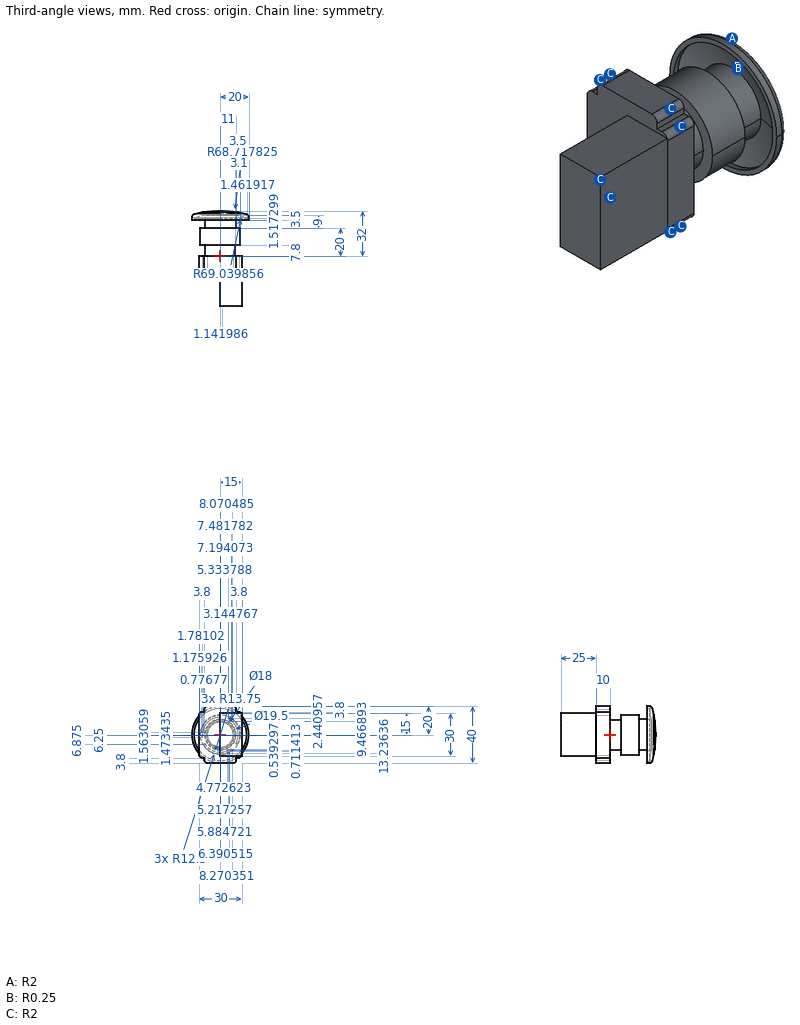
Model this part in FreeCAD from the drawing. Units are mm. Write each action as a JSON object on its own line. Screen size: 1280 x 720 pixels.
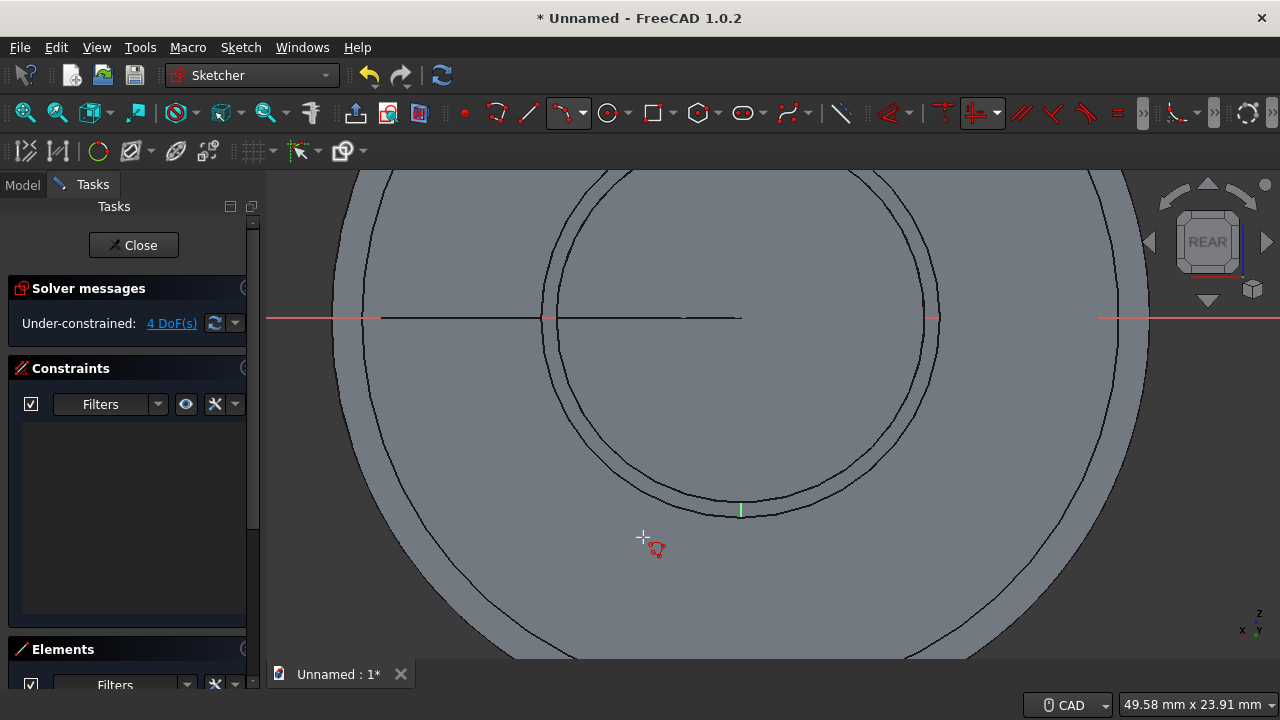
{"action": "left_click", "coordinate": [643, 536]}
{"action": "left_click", "coordinate": [571, 525]}
{"action": "left_click", "coordinate": [610, 589]}
{"action": "left_click", "coordinate": [620, 573]}
{"action": "right_click", "coordinate": [620, 573]}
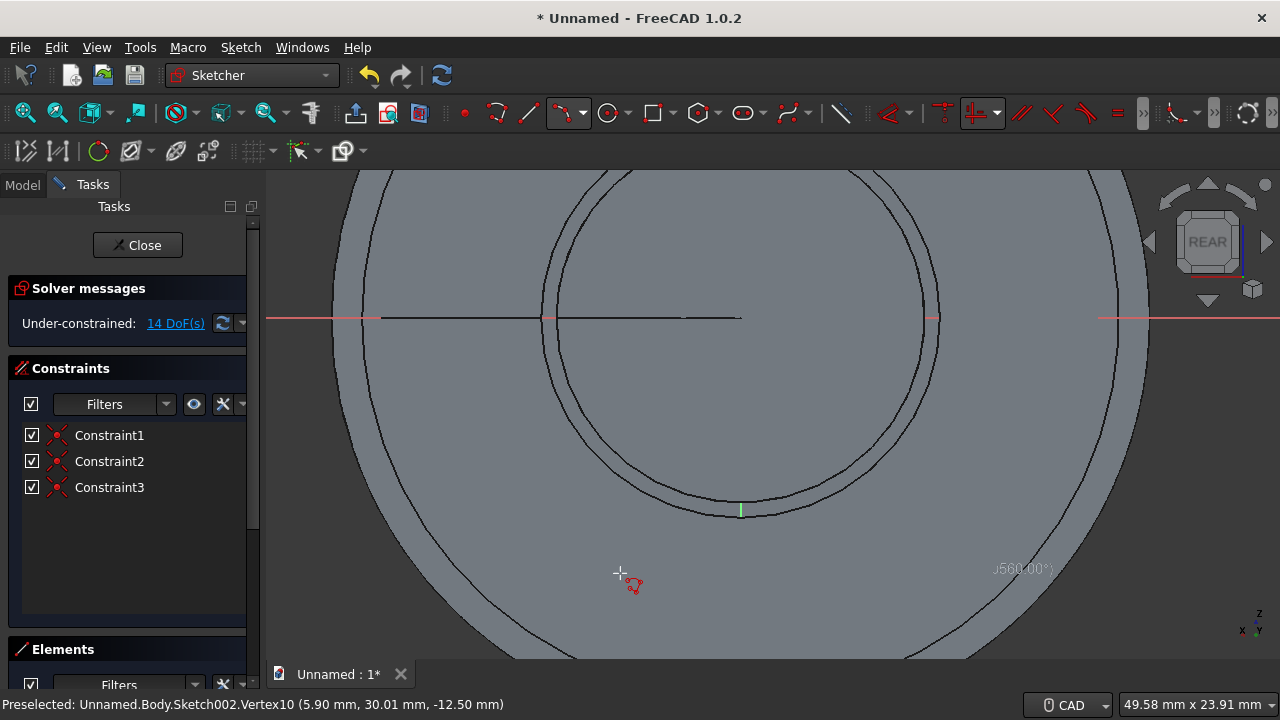
{"action": "left_click", "coordinate": [562, 114]}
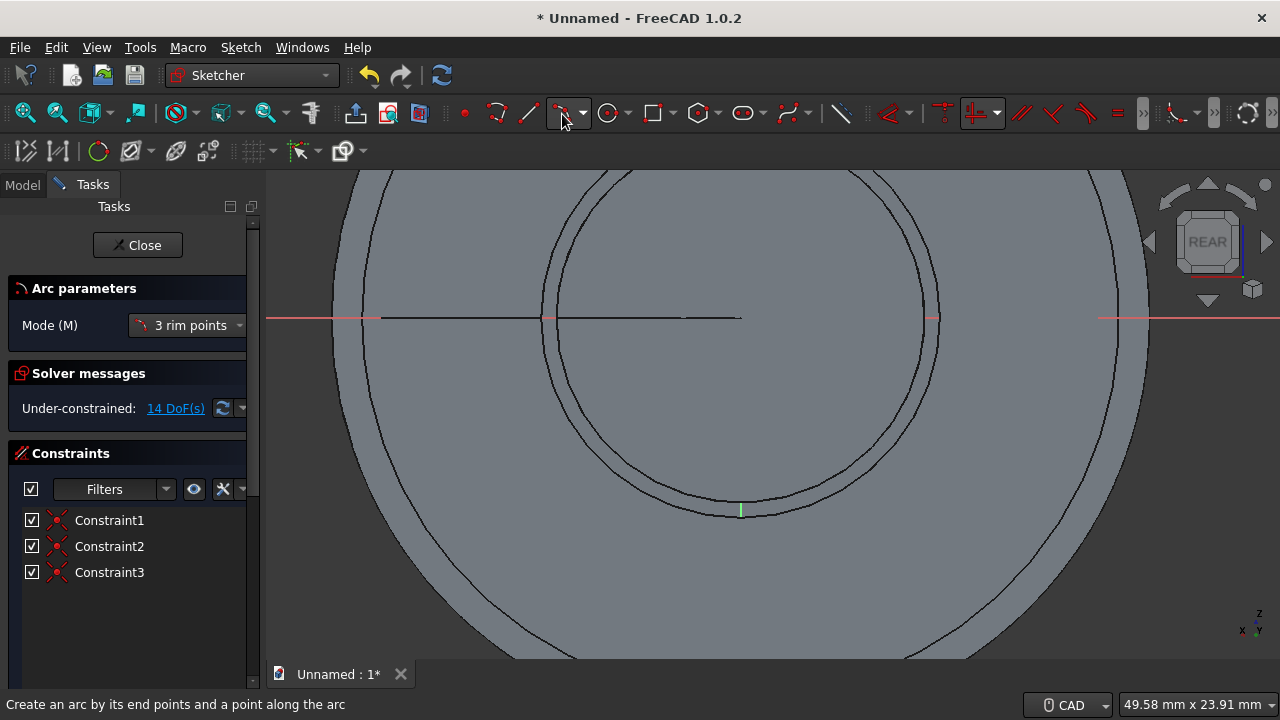
{"action": "scroll", "coordinate": [962, 446], "scroll_direction": "up", "scroll_amount": 2}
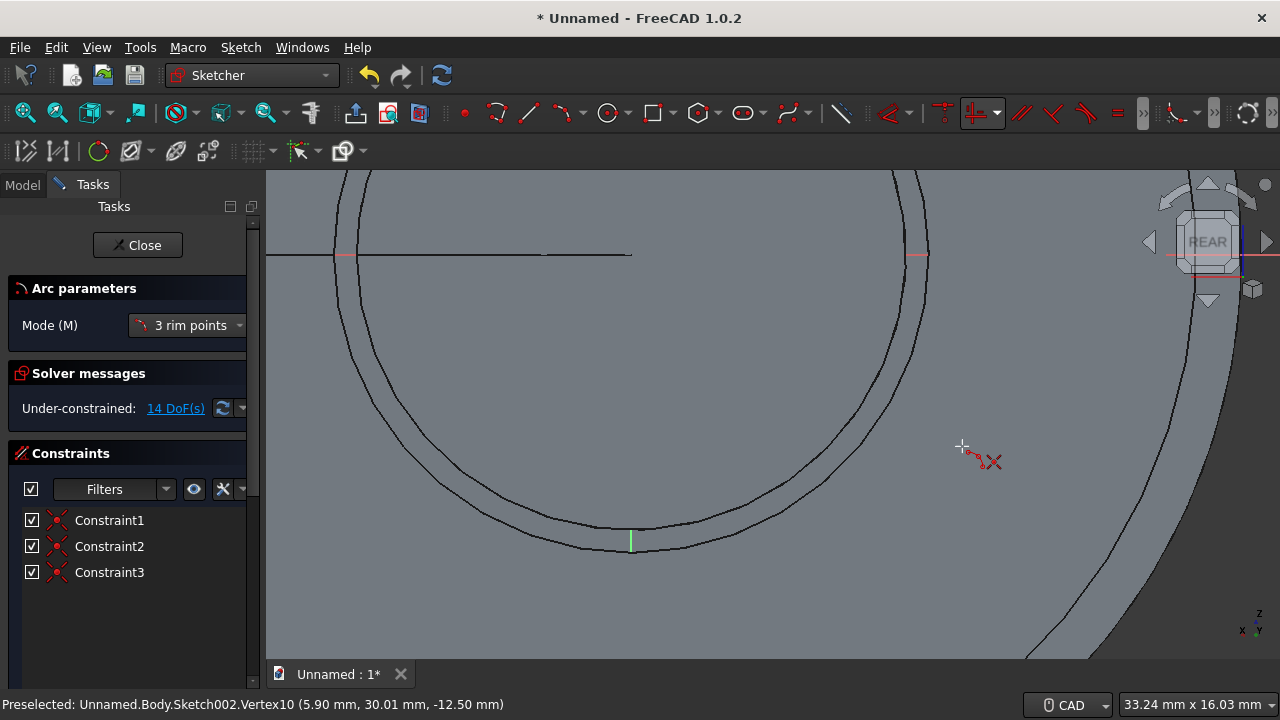
{"action": "left_click", "coordinate": [961, 450]}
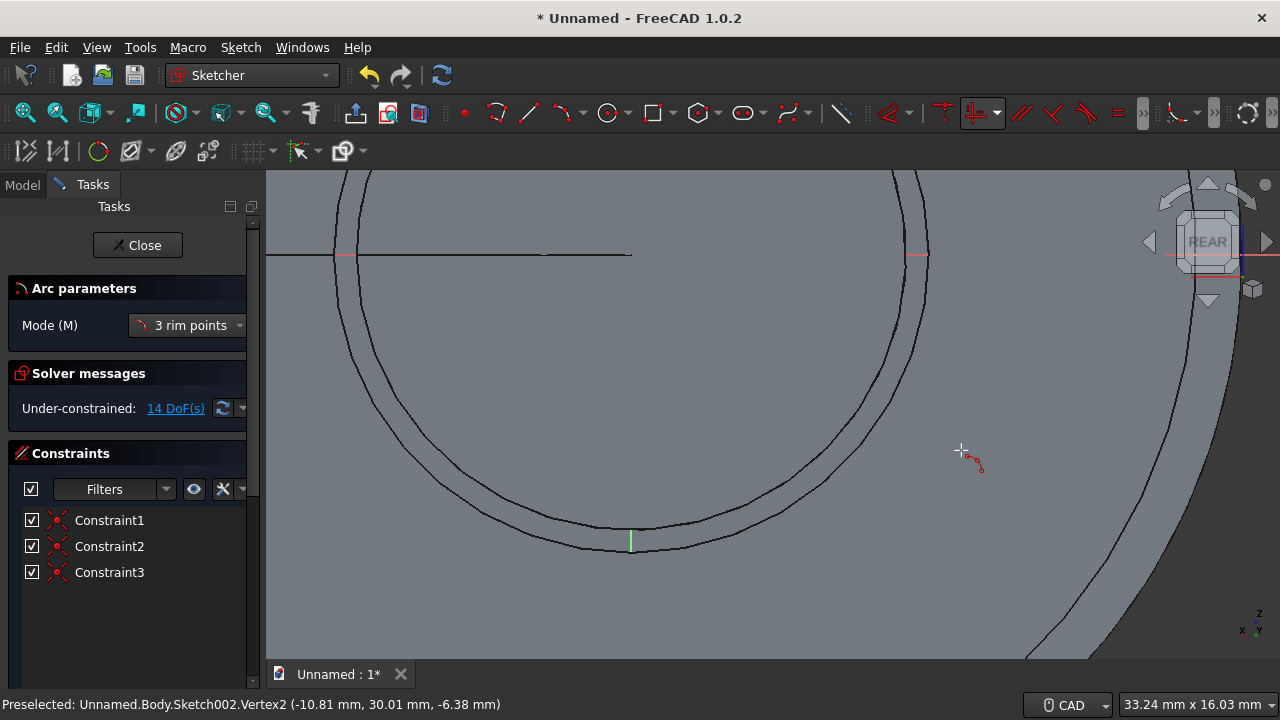
{"action": "scroll", "coordinate": [472, 602], "scroll_direction": "up", "scroll_amount": 2}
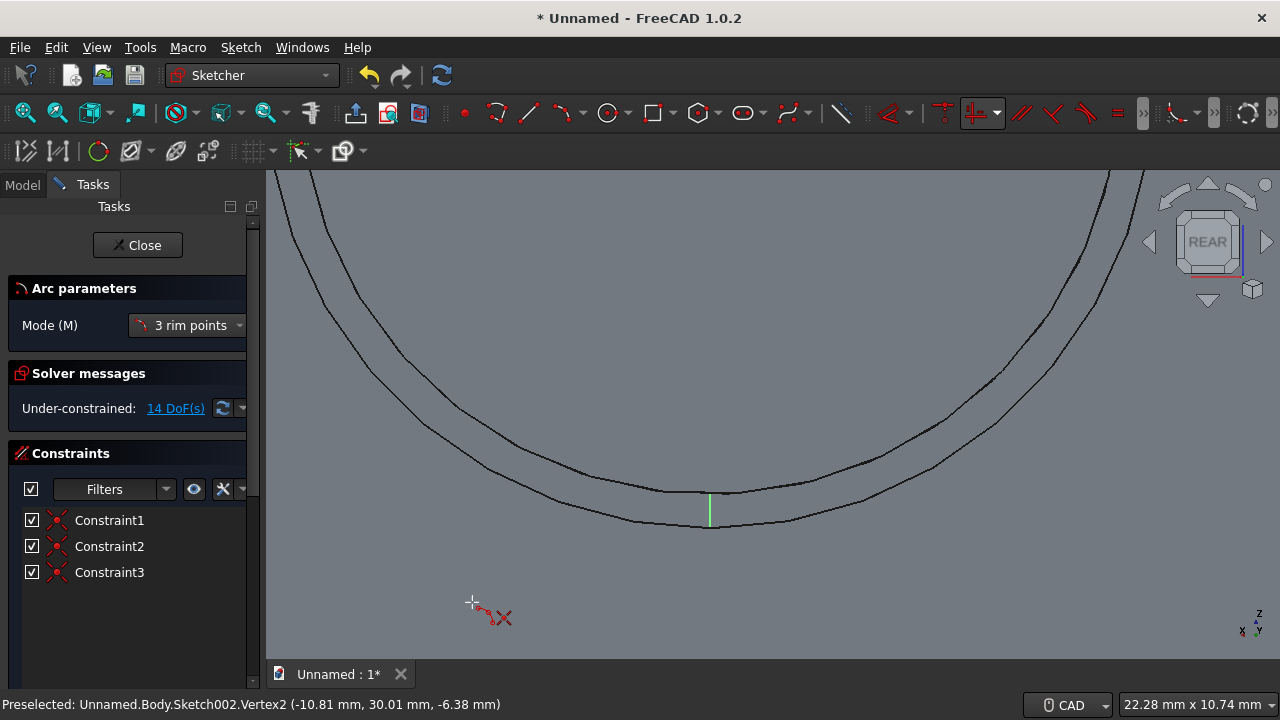
{"action": "left_click", "coordinate": [471, 606]}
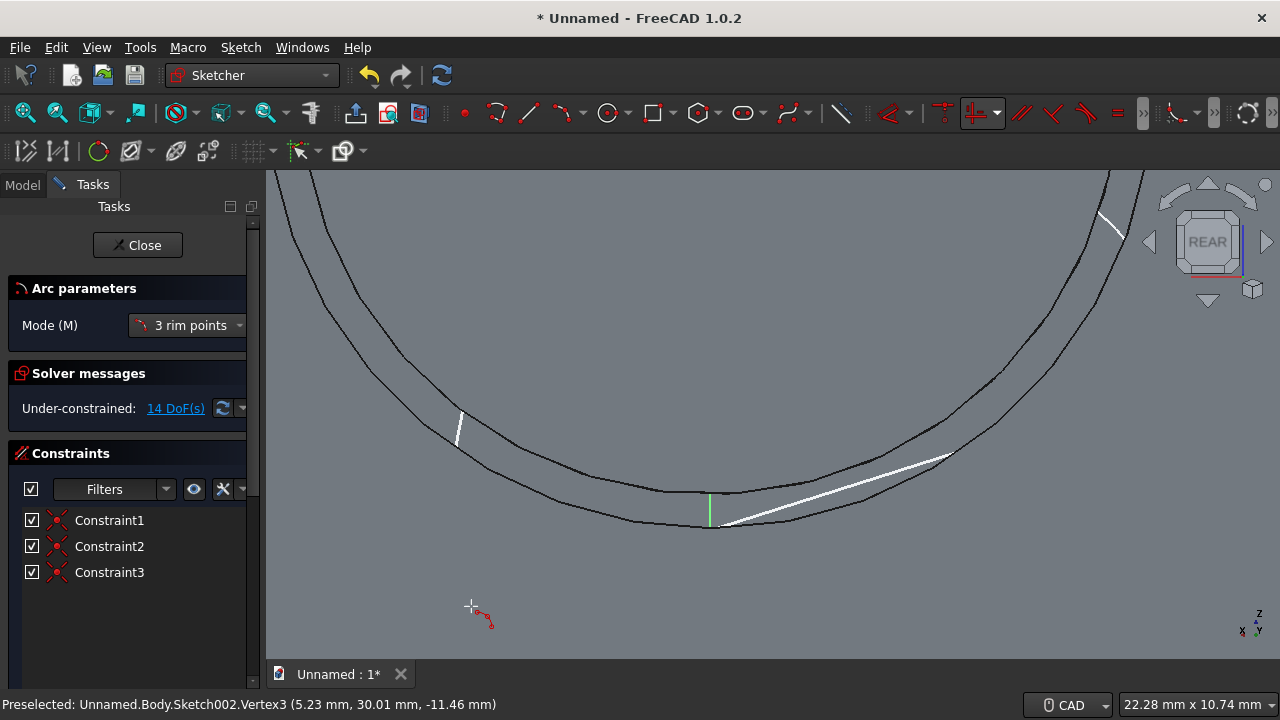
{"action": "scroll", "coordinate": [692, 526], "scroll_direction": "down", "scroll_amount": 7}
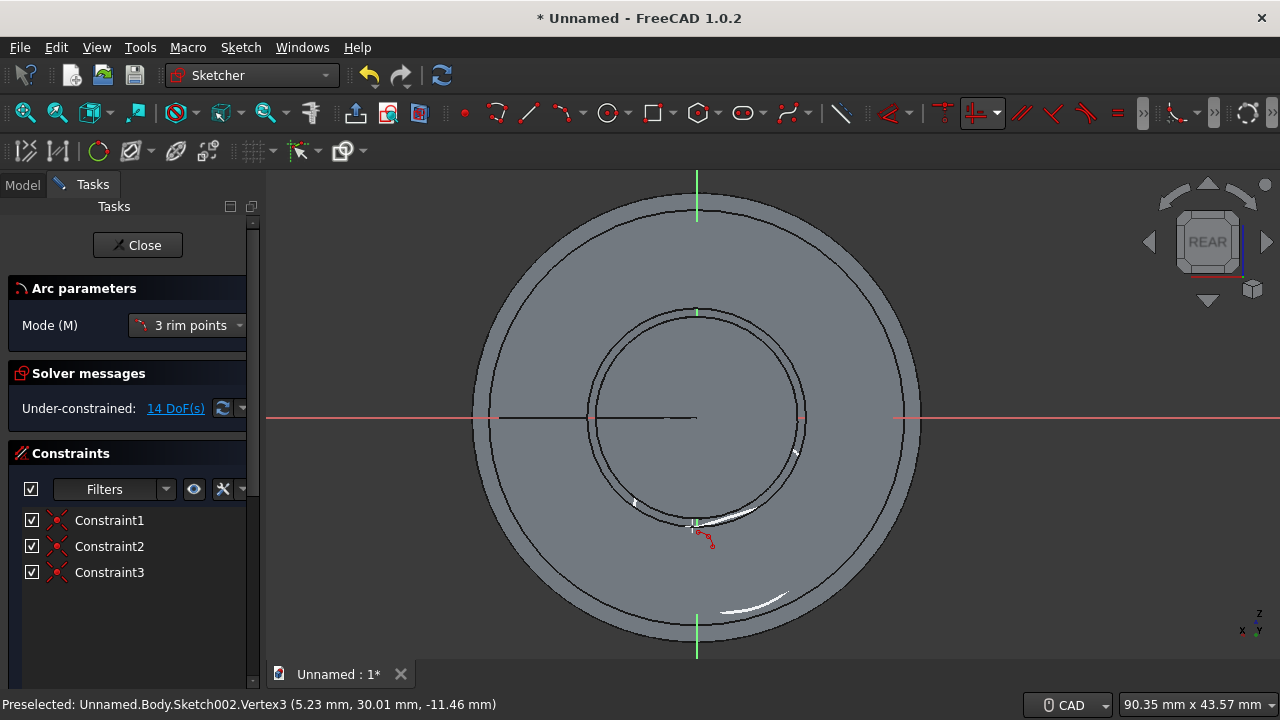
{"action": "left_click", "coordinate": [739, 551]}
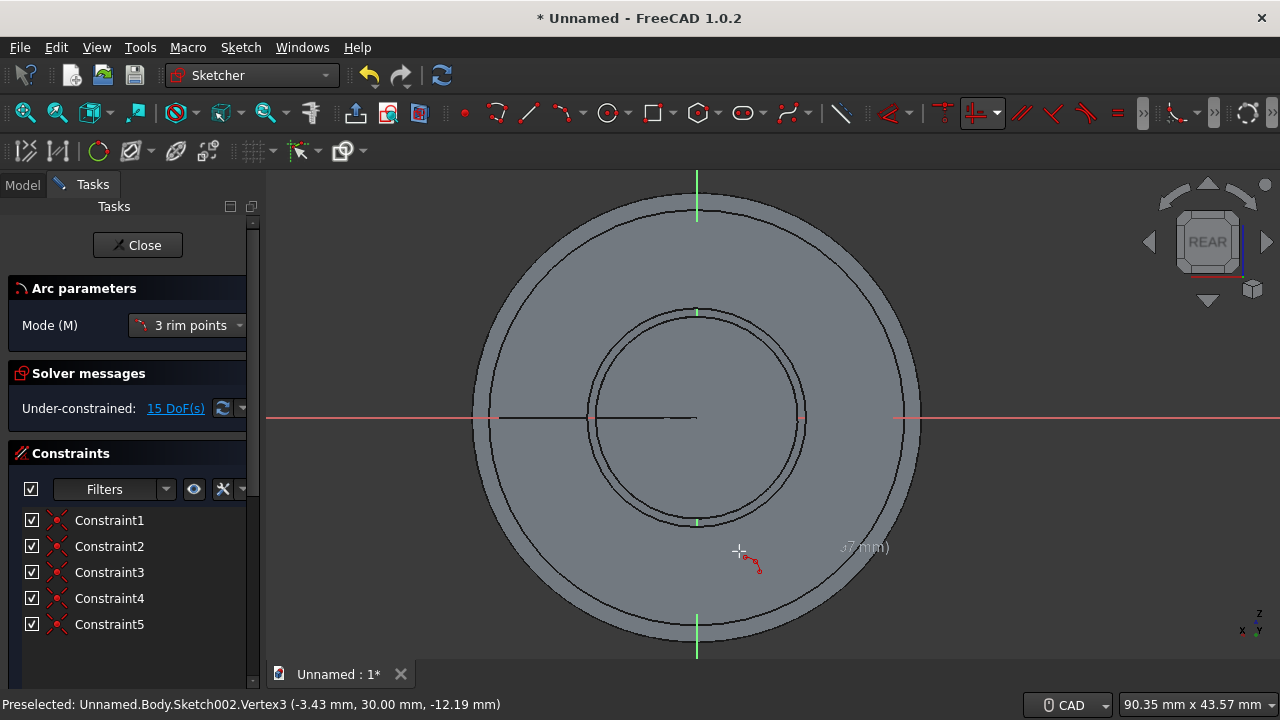
{"action": "scroll", "coordinate": [631, 557], "scroll_direction": "up", "scroll_amount": 6}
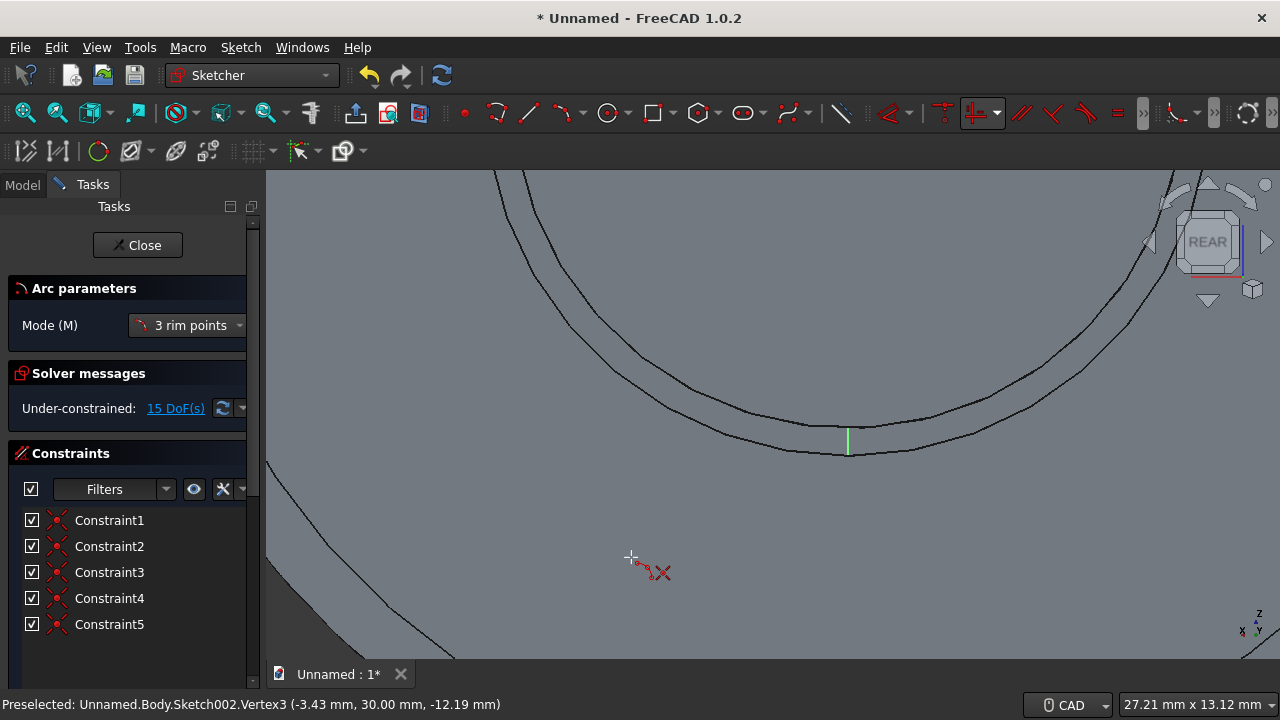
{"action": "left_click", "coordinate": [628, 558]}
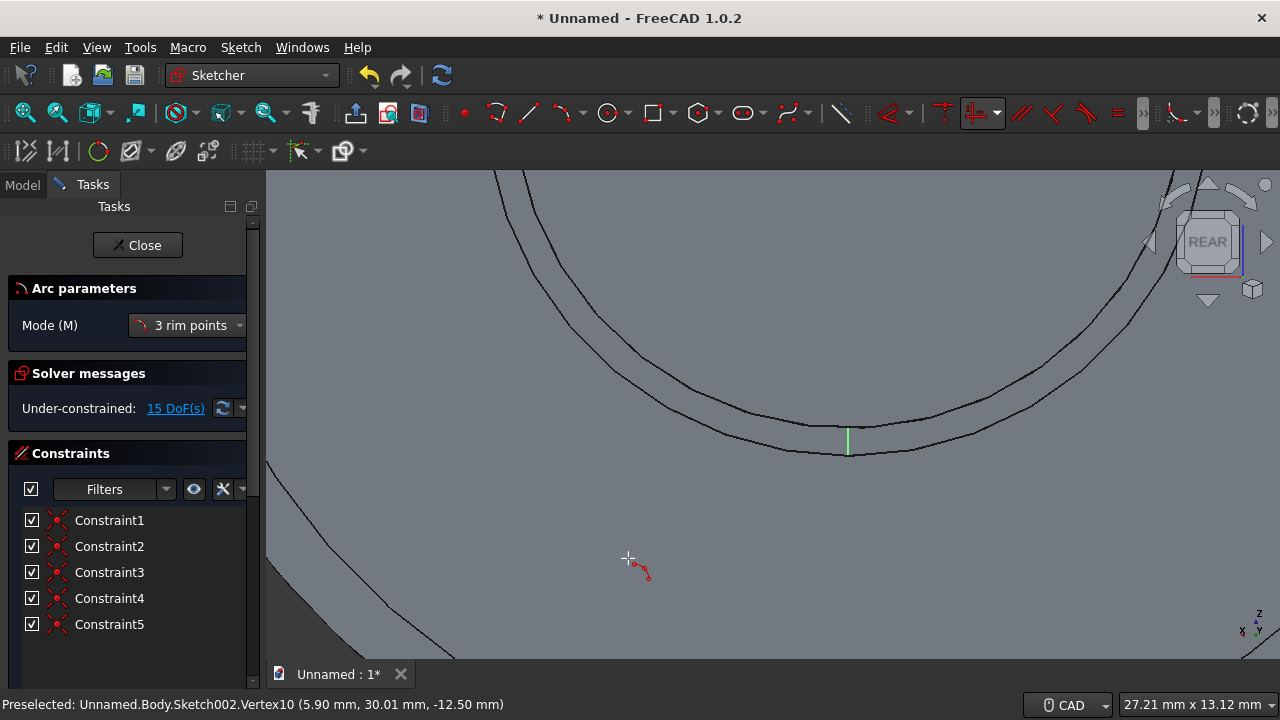
{"action": "scroll", "coordinate": [631, 557], "scroll_direction": "down", "scroll_amount": 6}